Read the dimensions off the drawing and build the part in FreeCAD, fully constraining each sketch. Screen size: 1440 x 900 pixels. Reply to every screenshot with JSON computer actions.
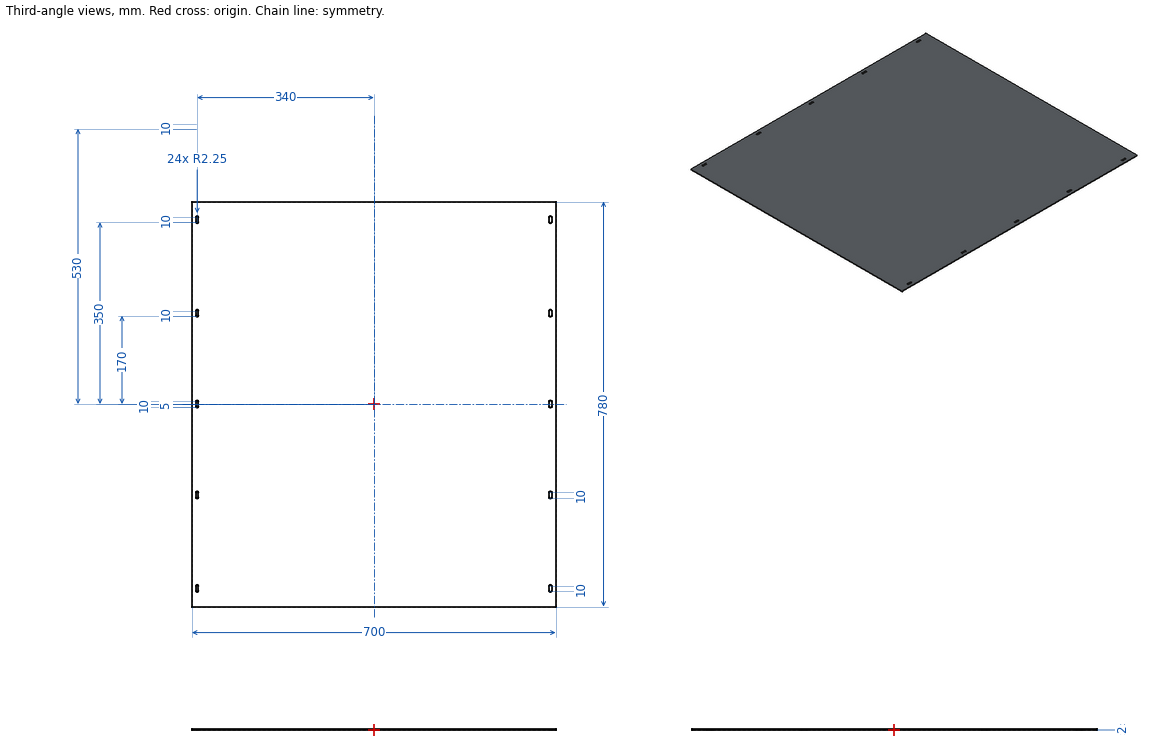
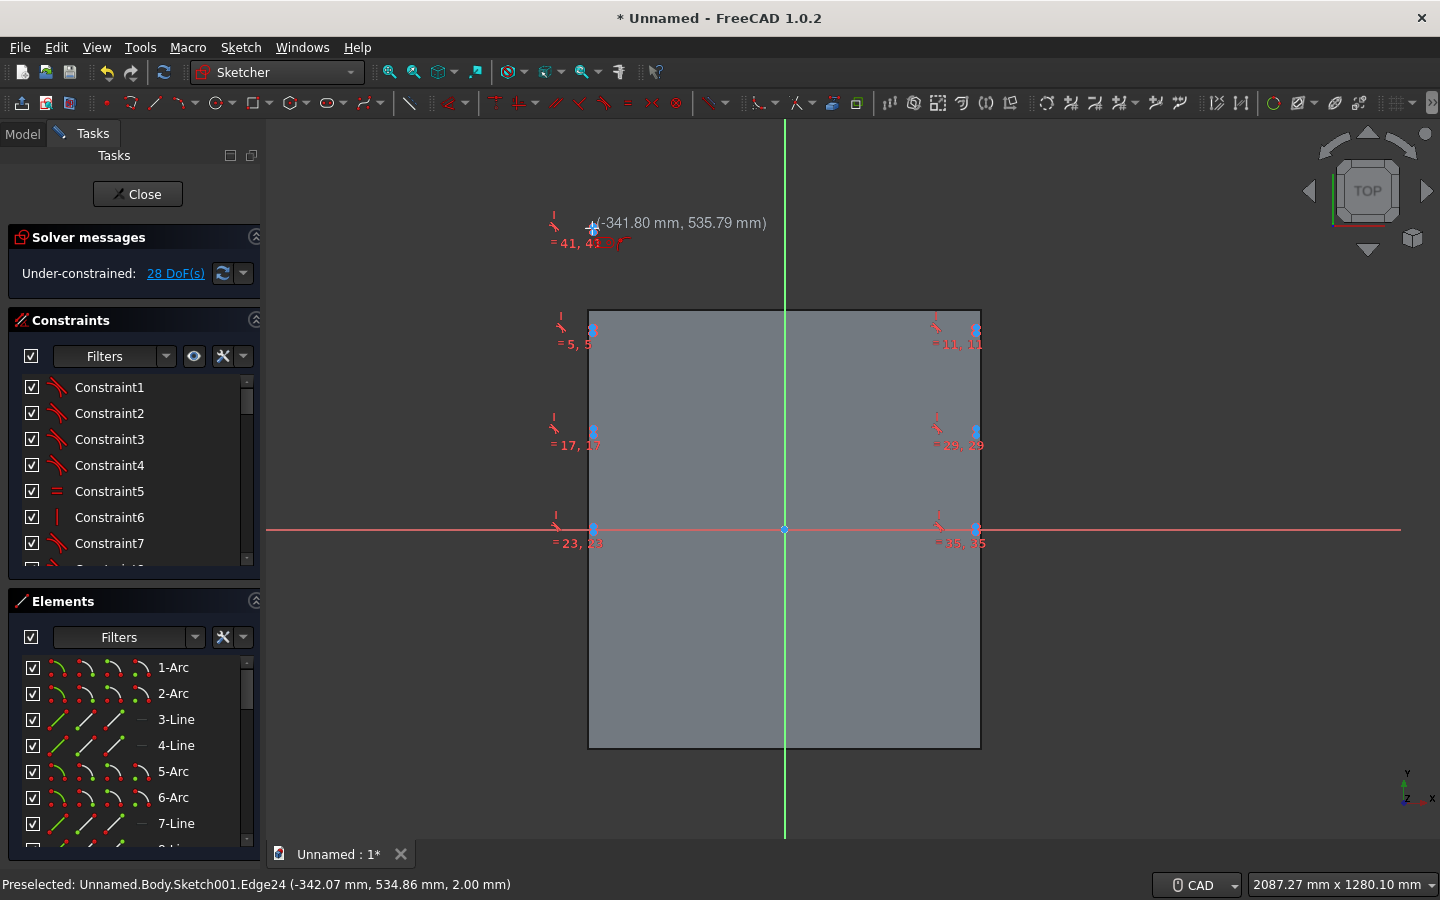
{"action": "scroll", "coordinate": [976, 231], "scroll_direction": "up", "scroll_amount": 15}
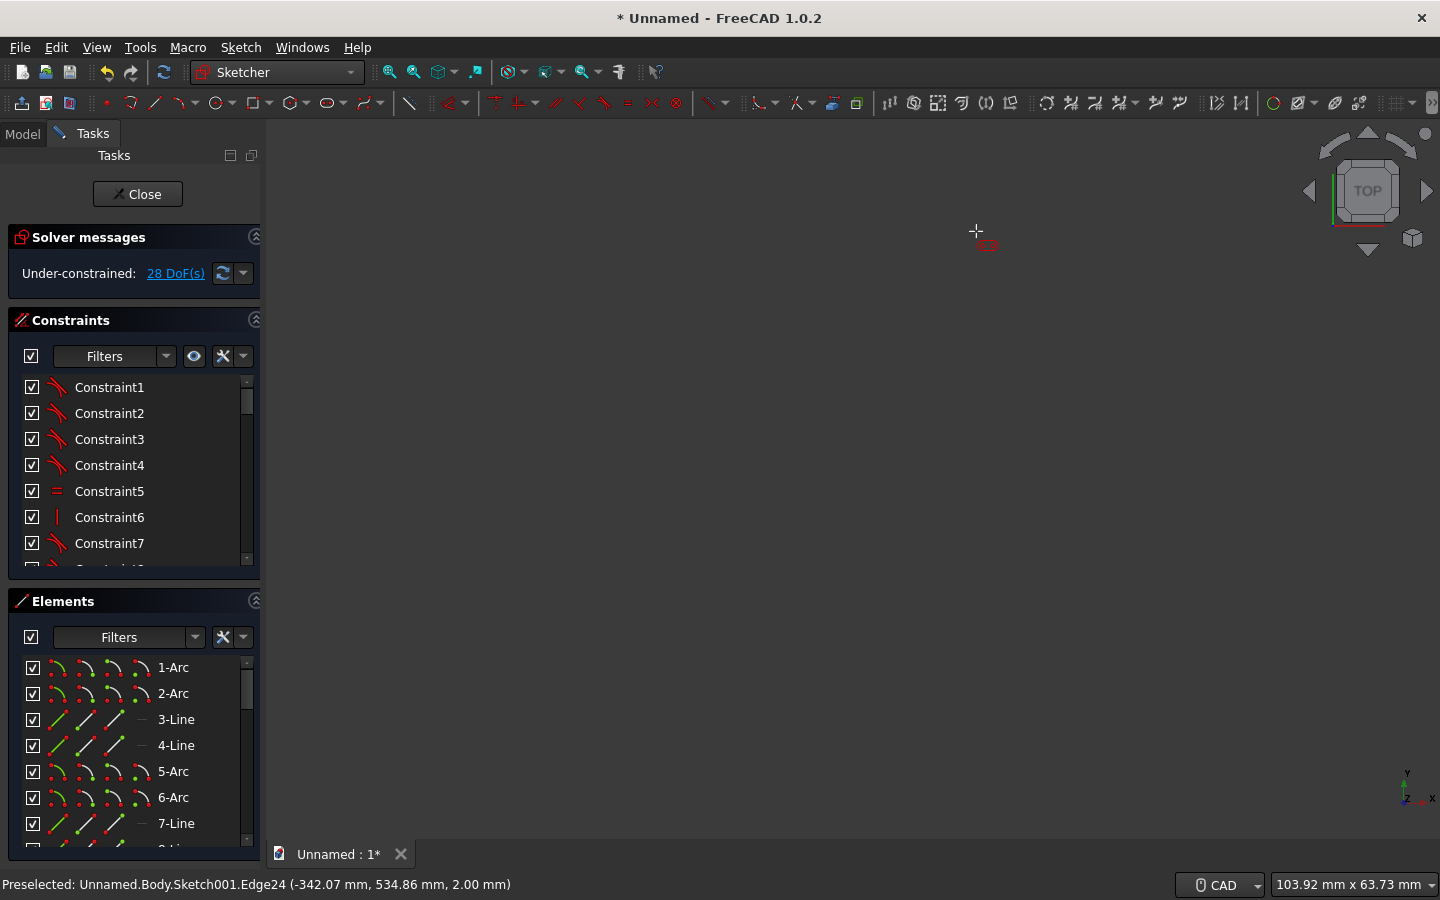
{"action": "scroll", "coordinate": [977, 231], "scroll_direction": "down", "scroll_amount": 15}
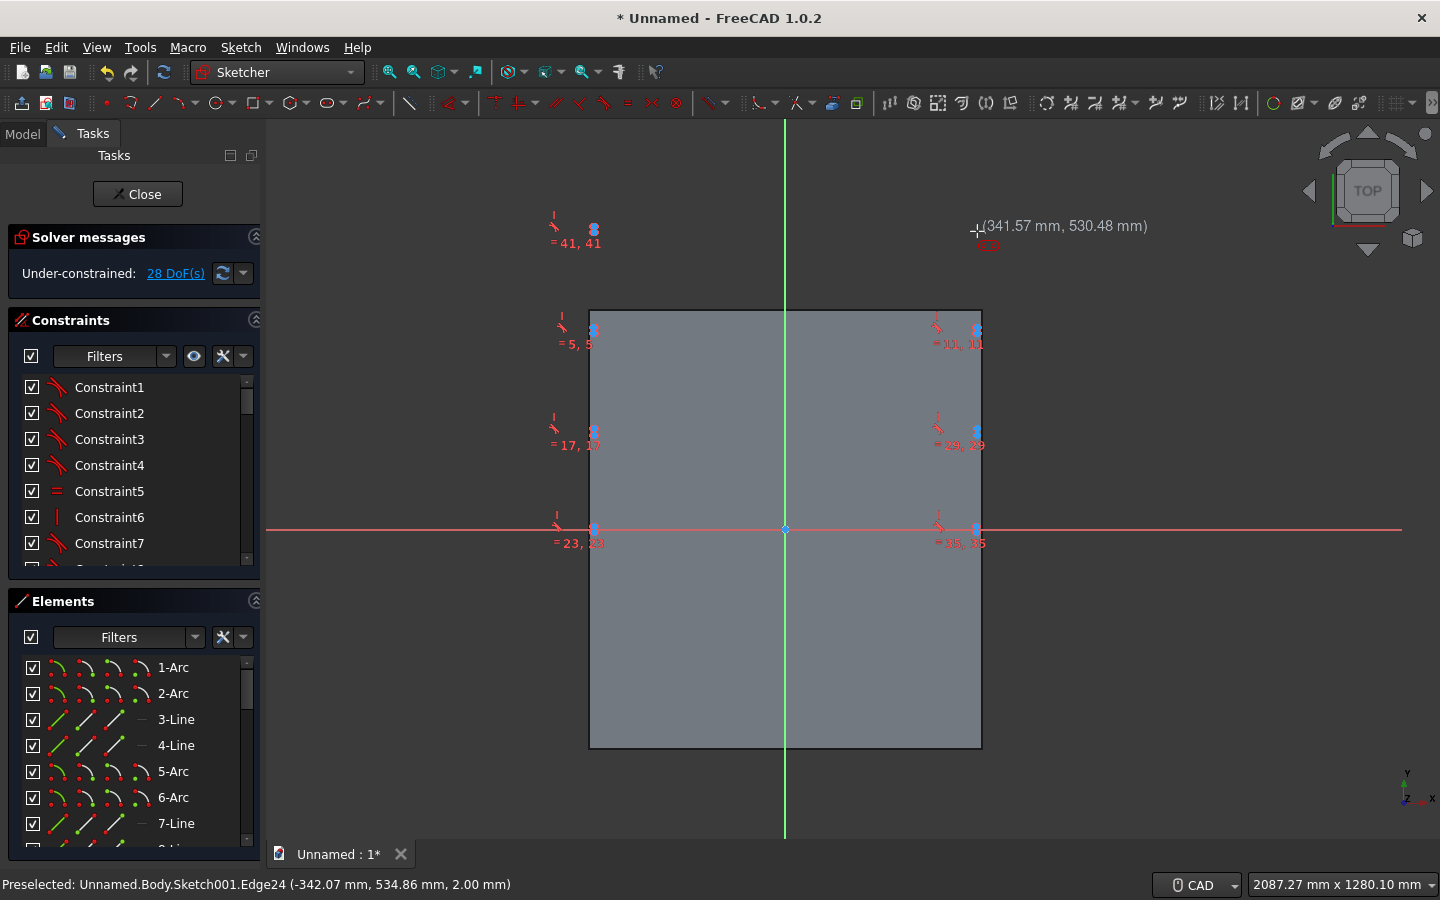
{"action": "left_click", "coordinate": [977, 231]}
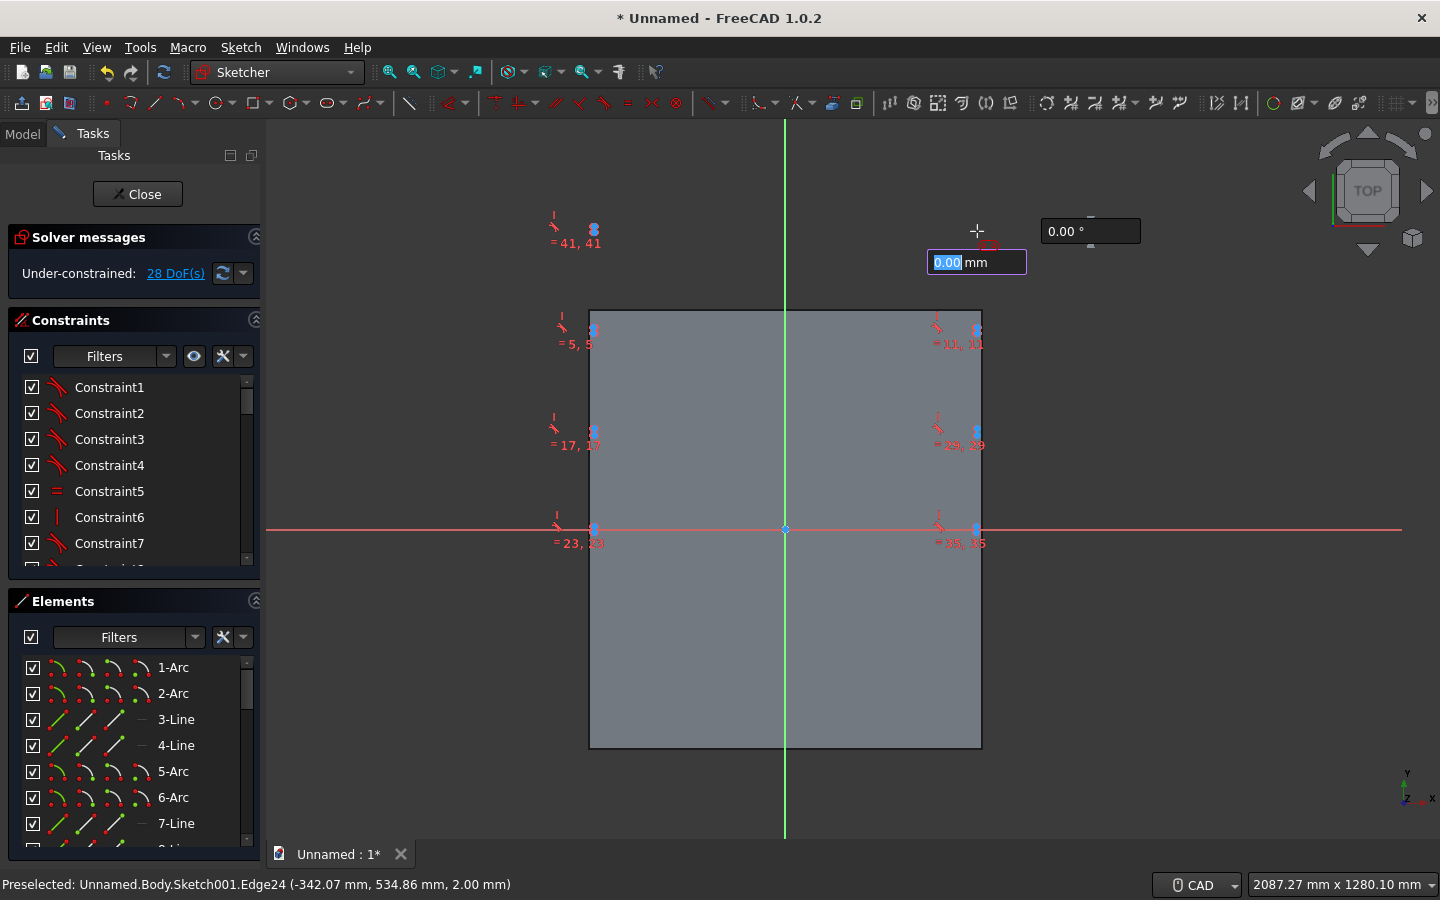
{"action": "scroll", "coordinate": [977, 226], "scroll_direction": "up", "scroll_amount": 6}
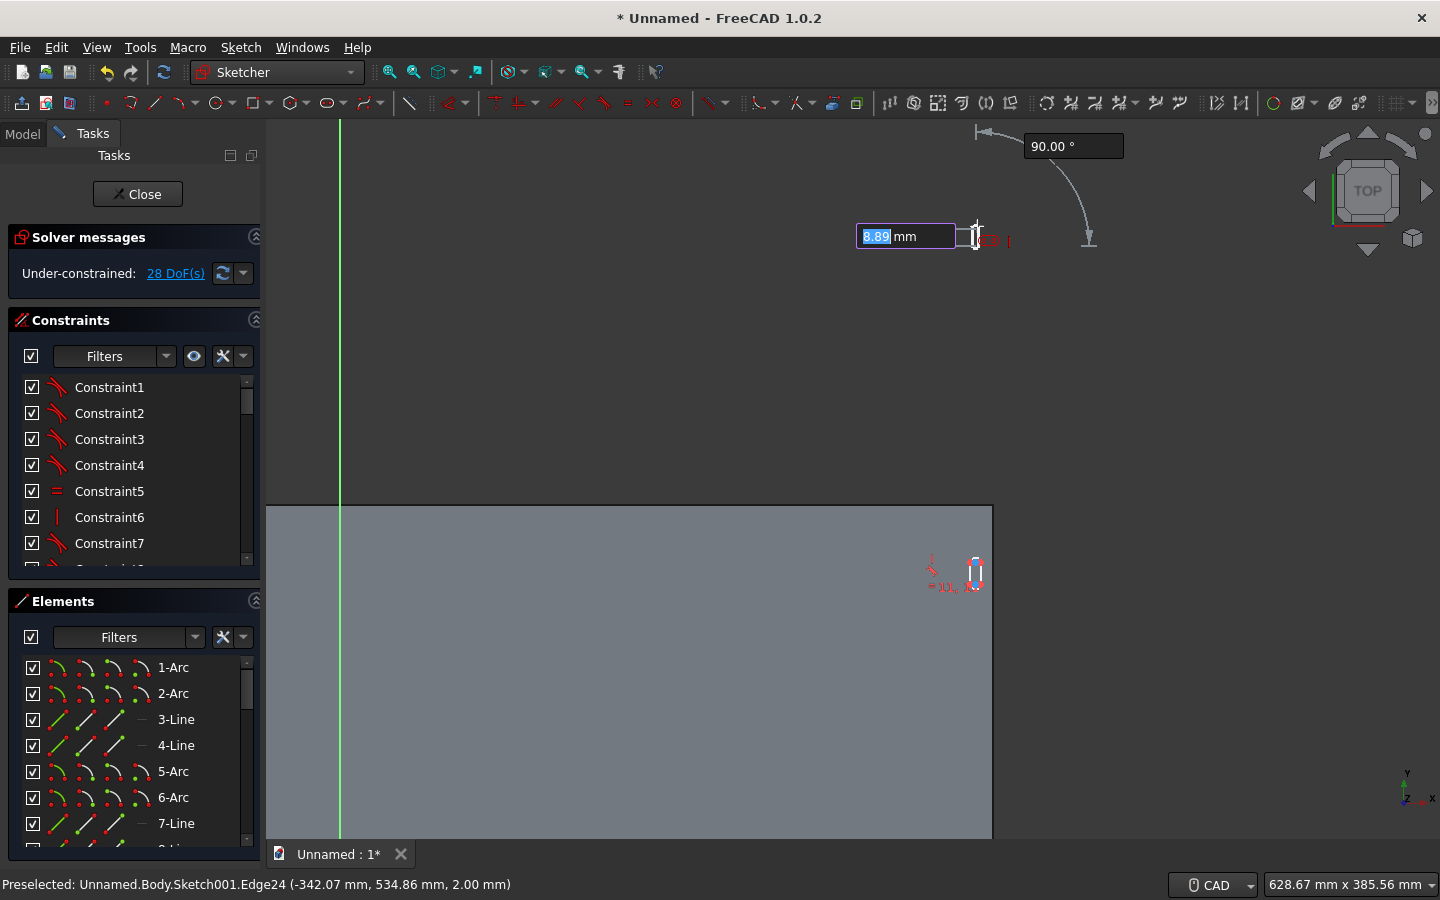
{"action": "left_click", "coordinate": [976, 225]}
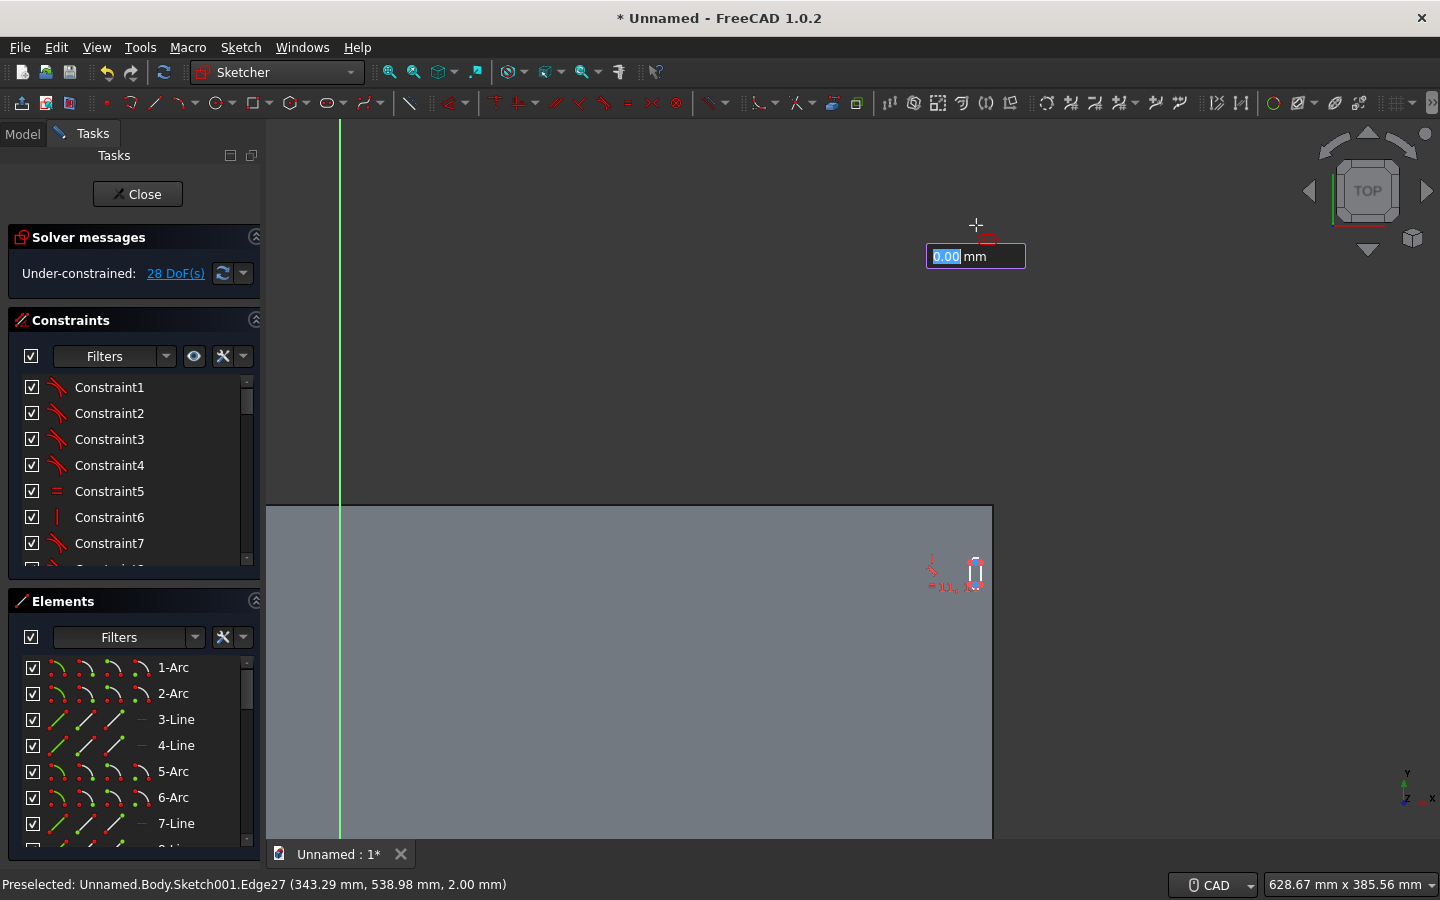
{"action": "scroll", "coordinate": [979, 234], "scroll_direction": "up", "scroll_amount": 7}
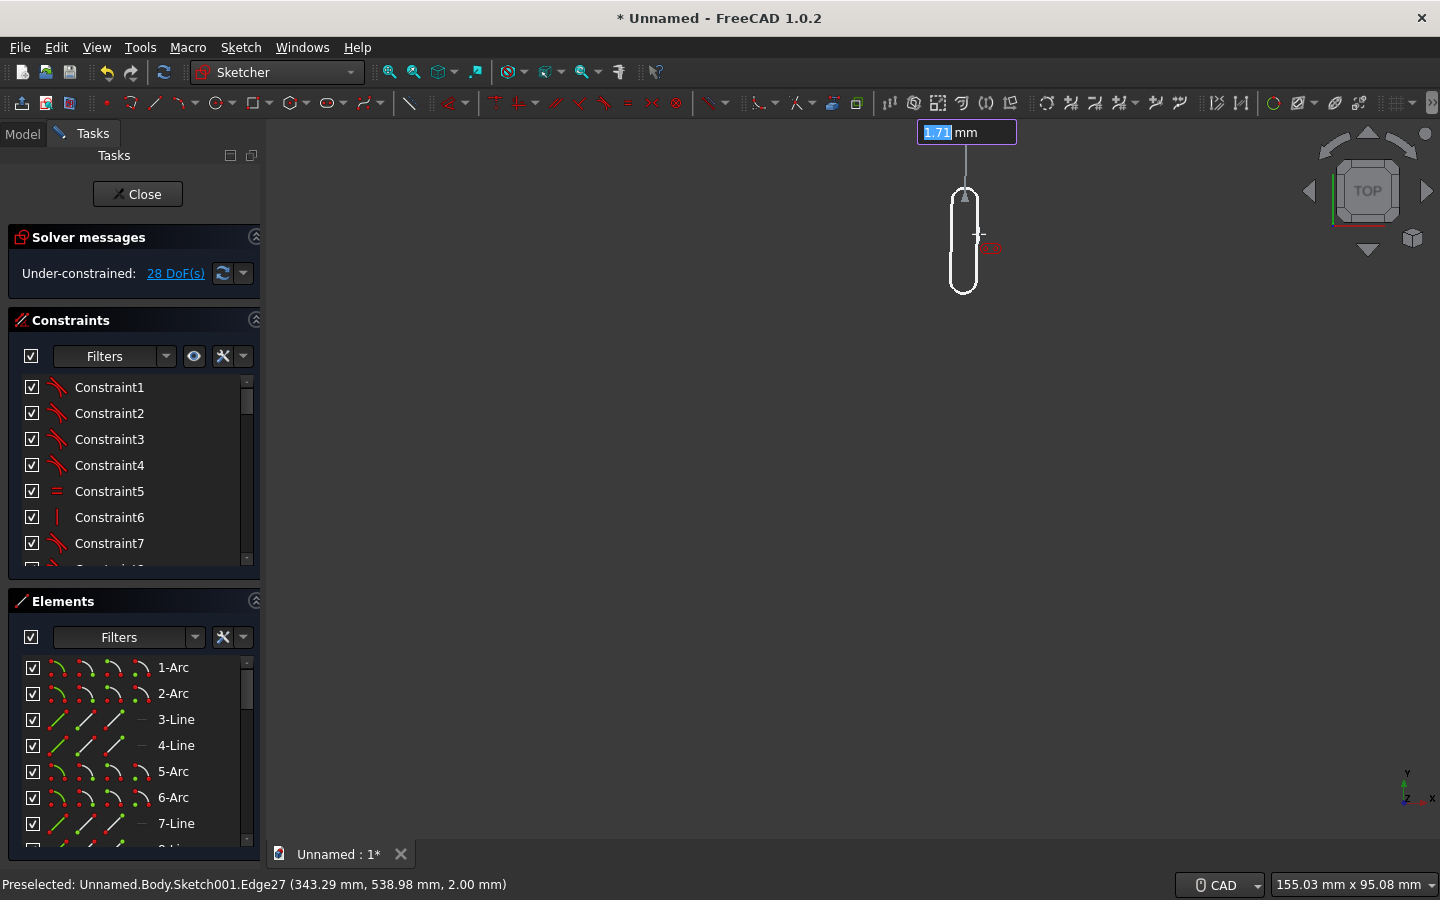
{"action": "left_click", "coordinate": [976, 235]}